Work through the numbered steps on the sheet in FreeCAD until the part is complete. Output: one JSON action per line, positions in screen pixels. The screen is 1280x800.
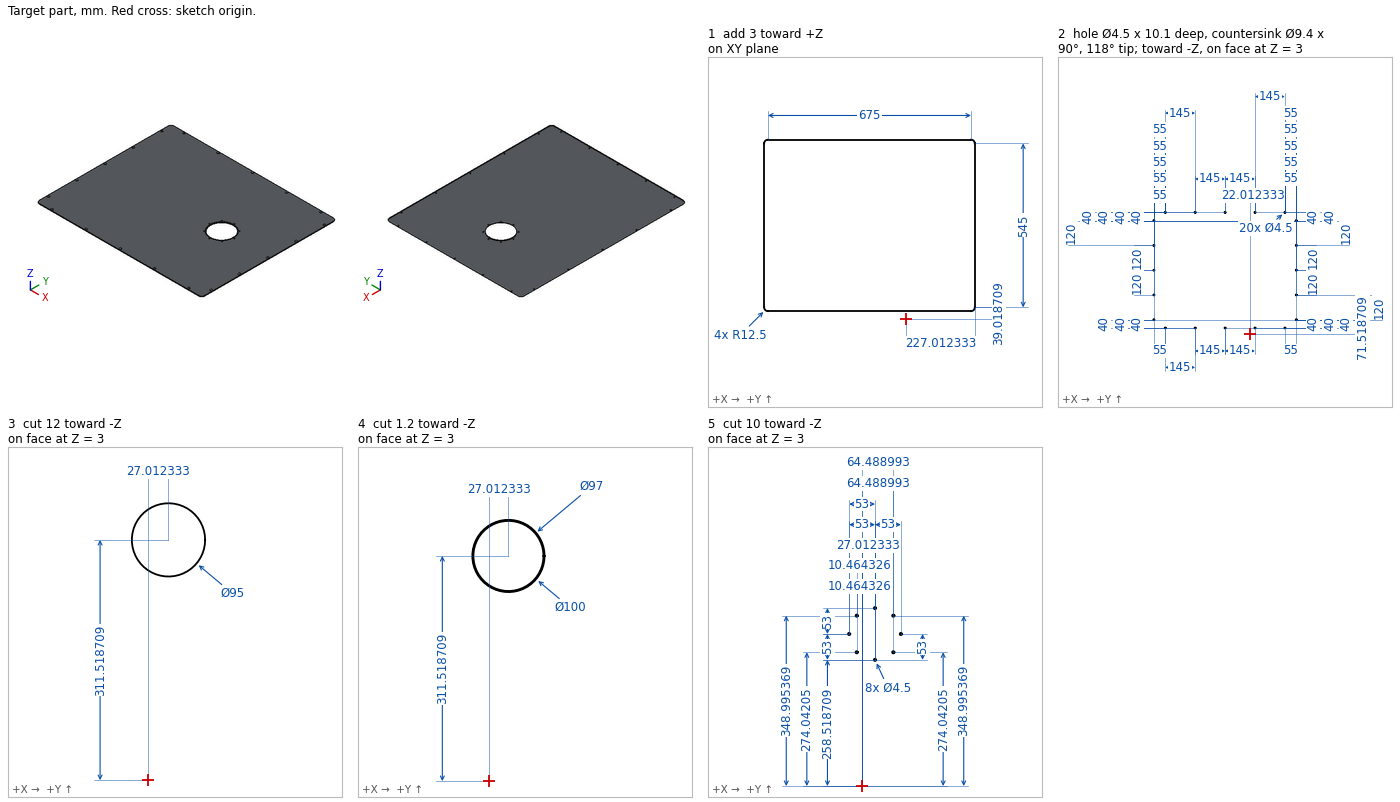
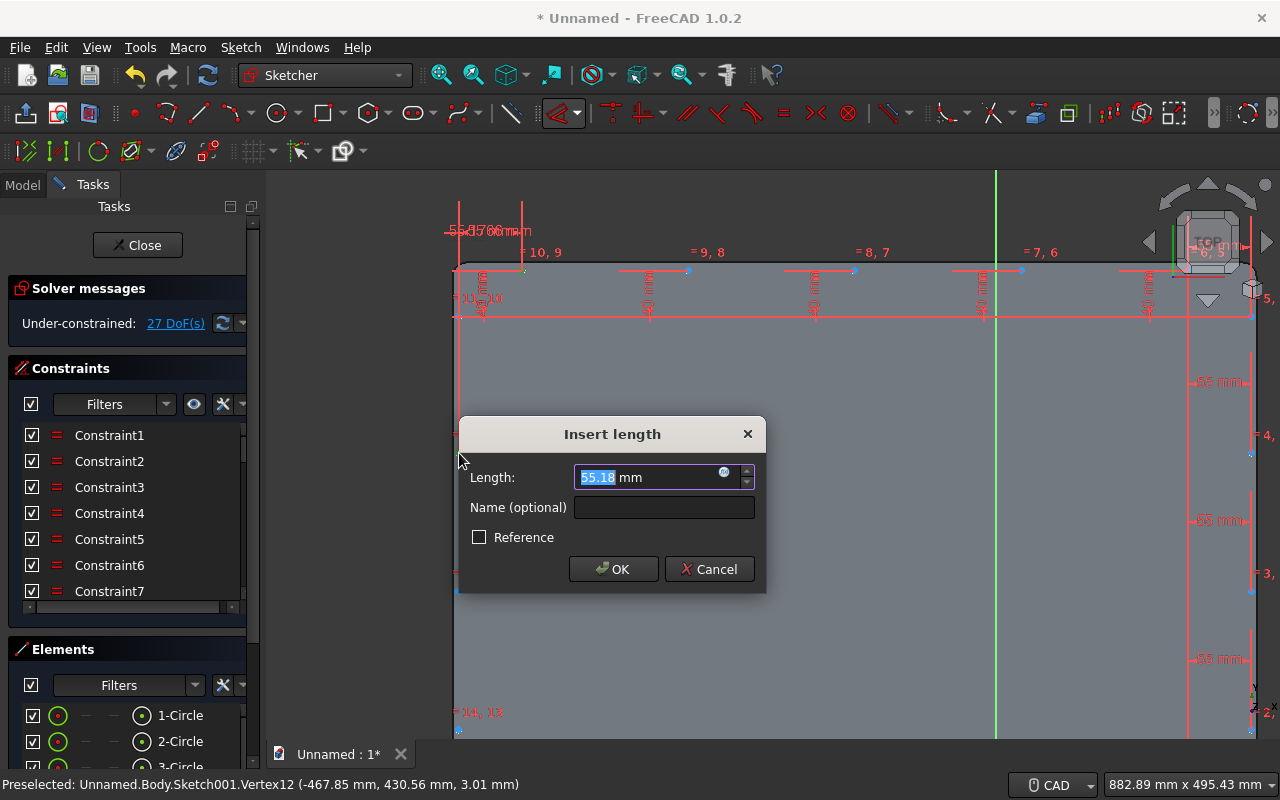
{"action": "type", "text": "55"}
{"action": "key", "text": "Return"}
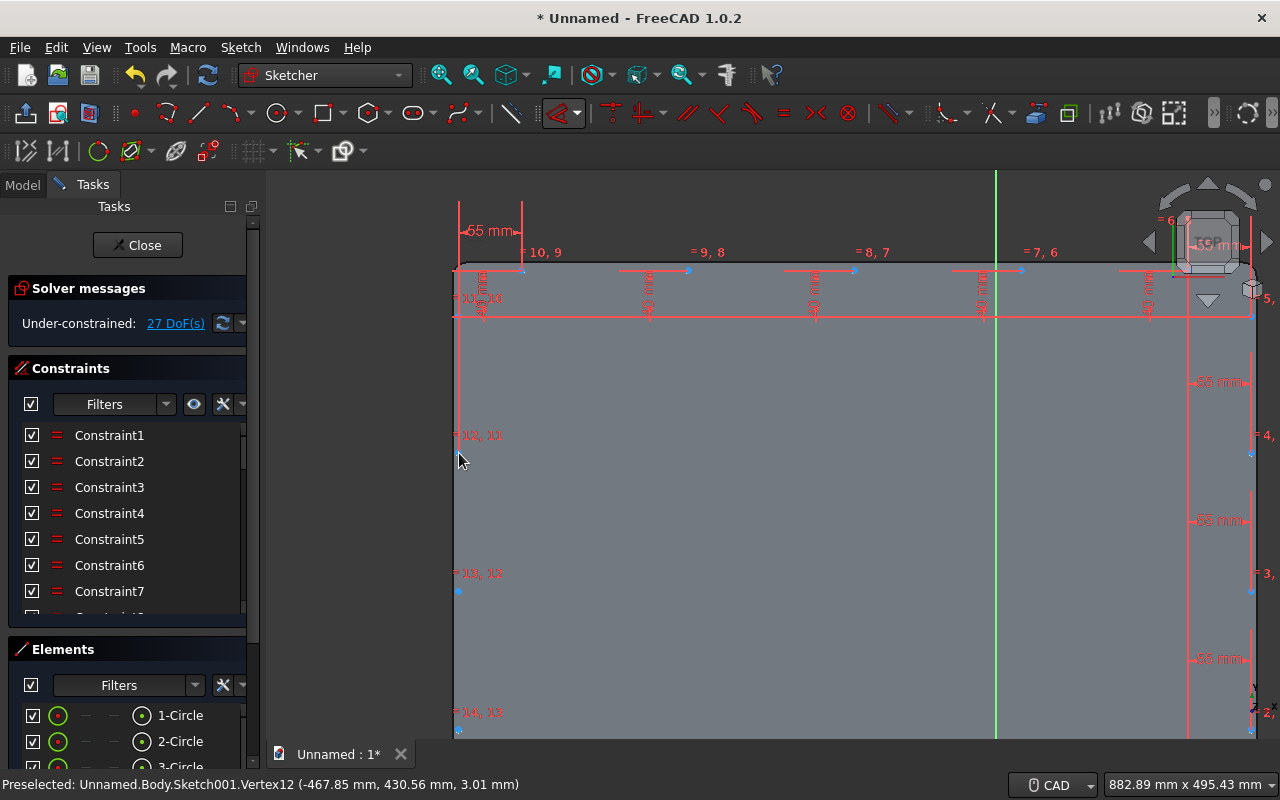
{"action": "left_click", "coordinate": [522, 271]}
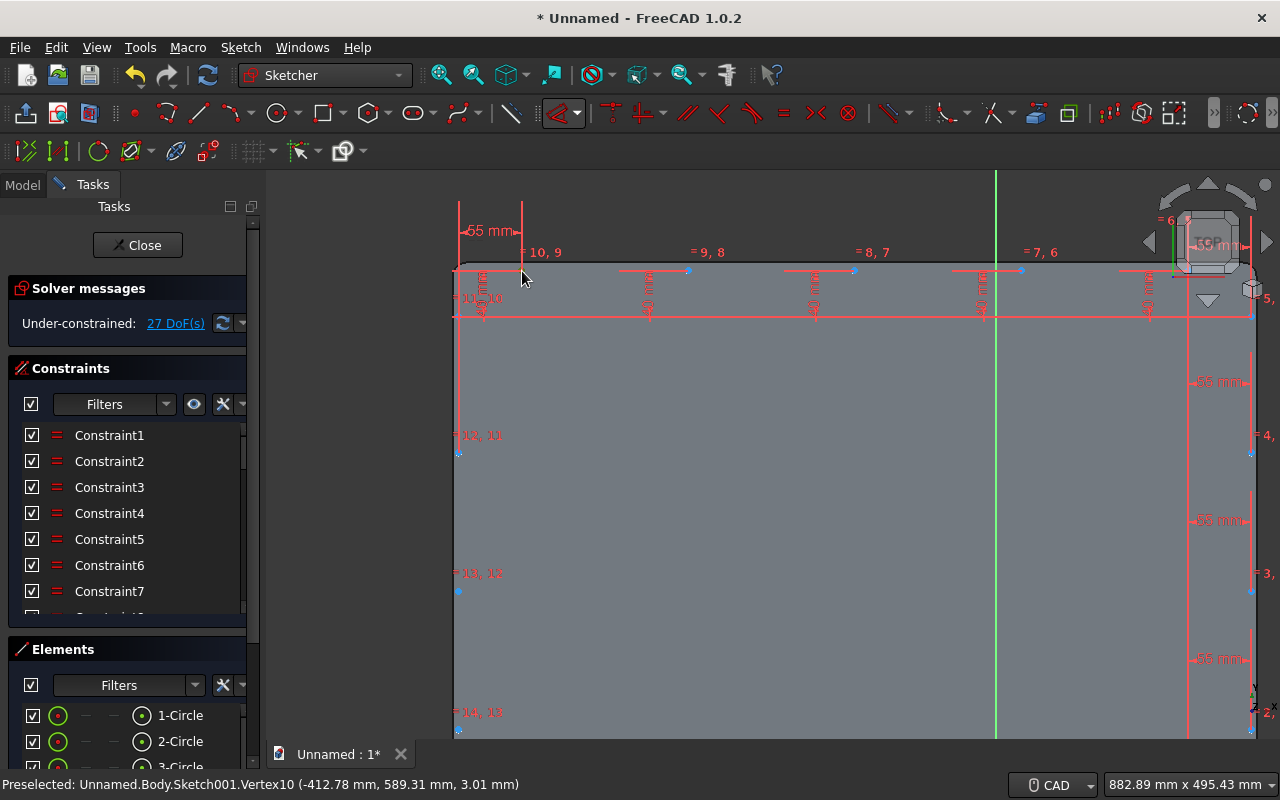
{"action": "left_click", "coordinate": [459, 591]}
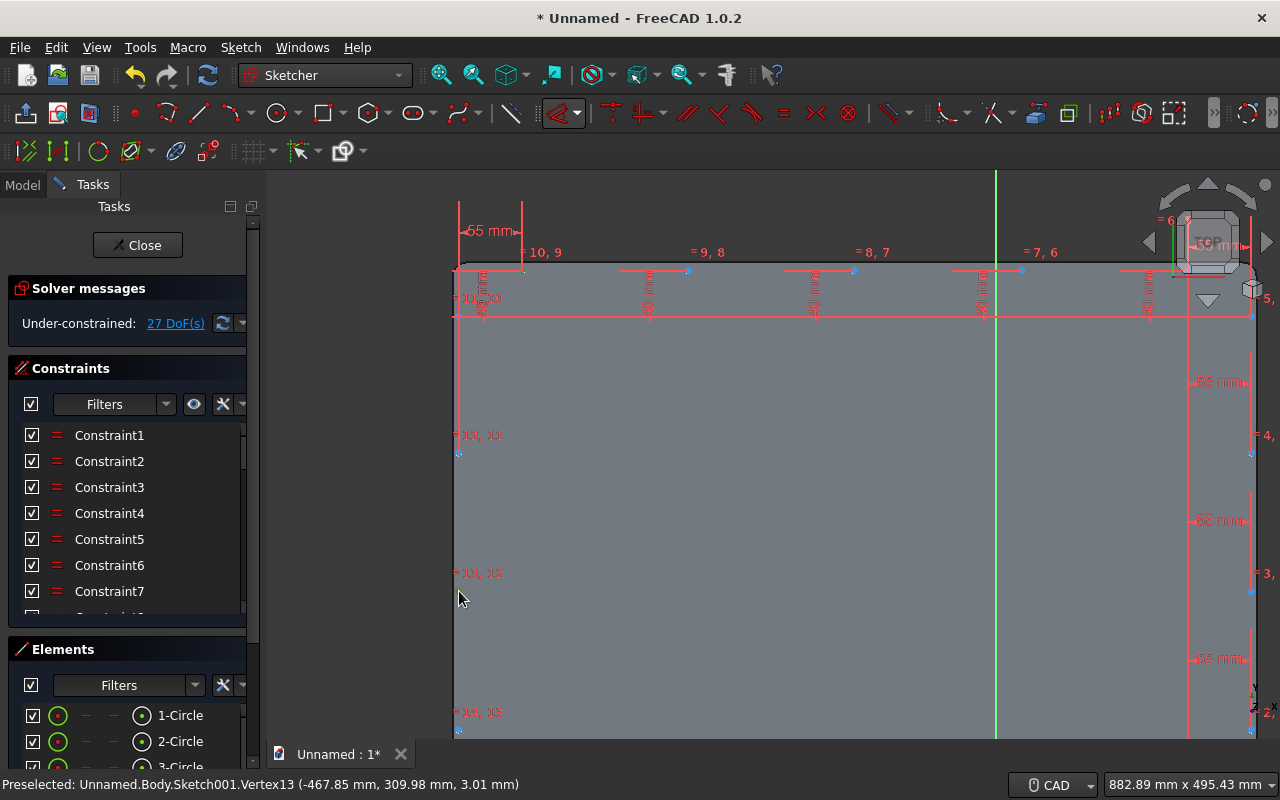
{"action": "left_click", "coordinate": [580, 114]}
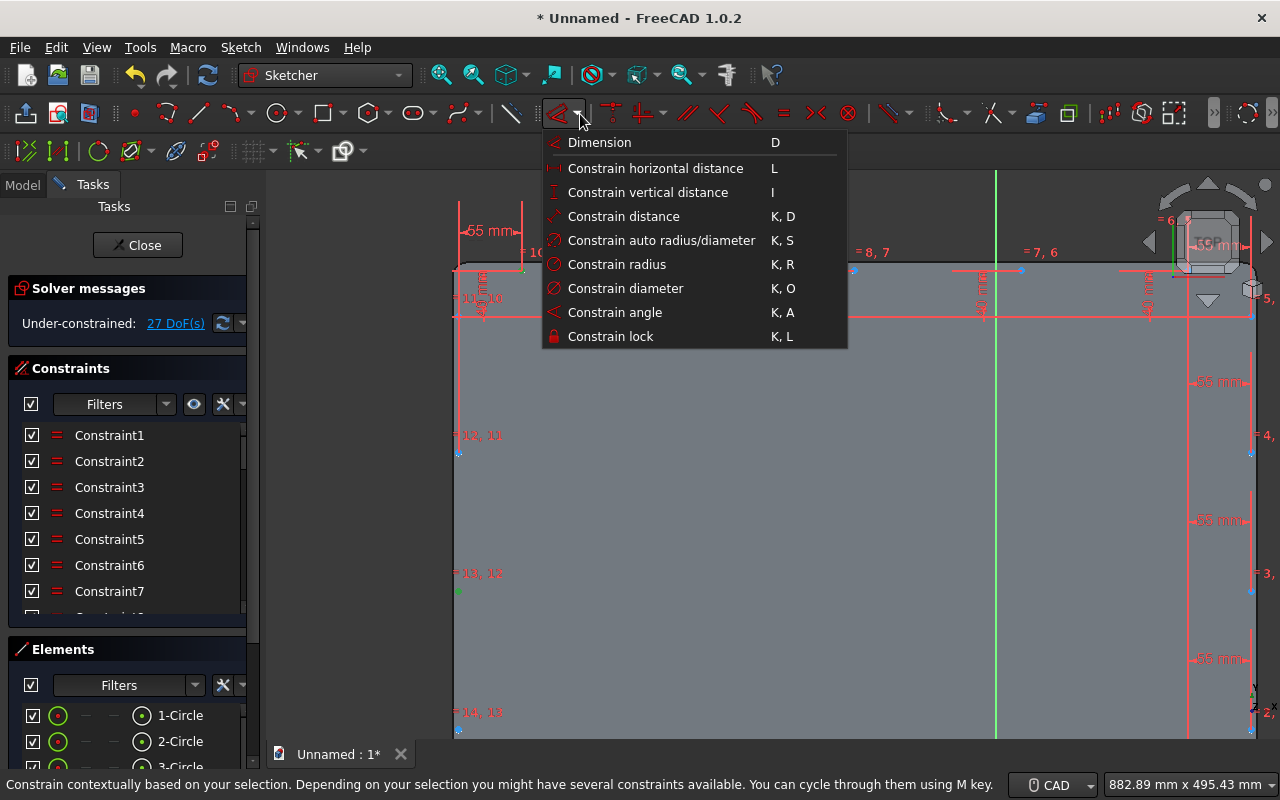
{"action": "left_click", "coordinate": [695, 168]}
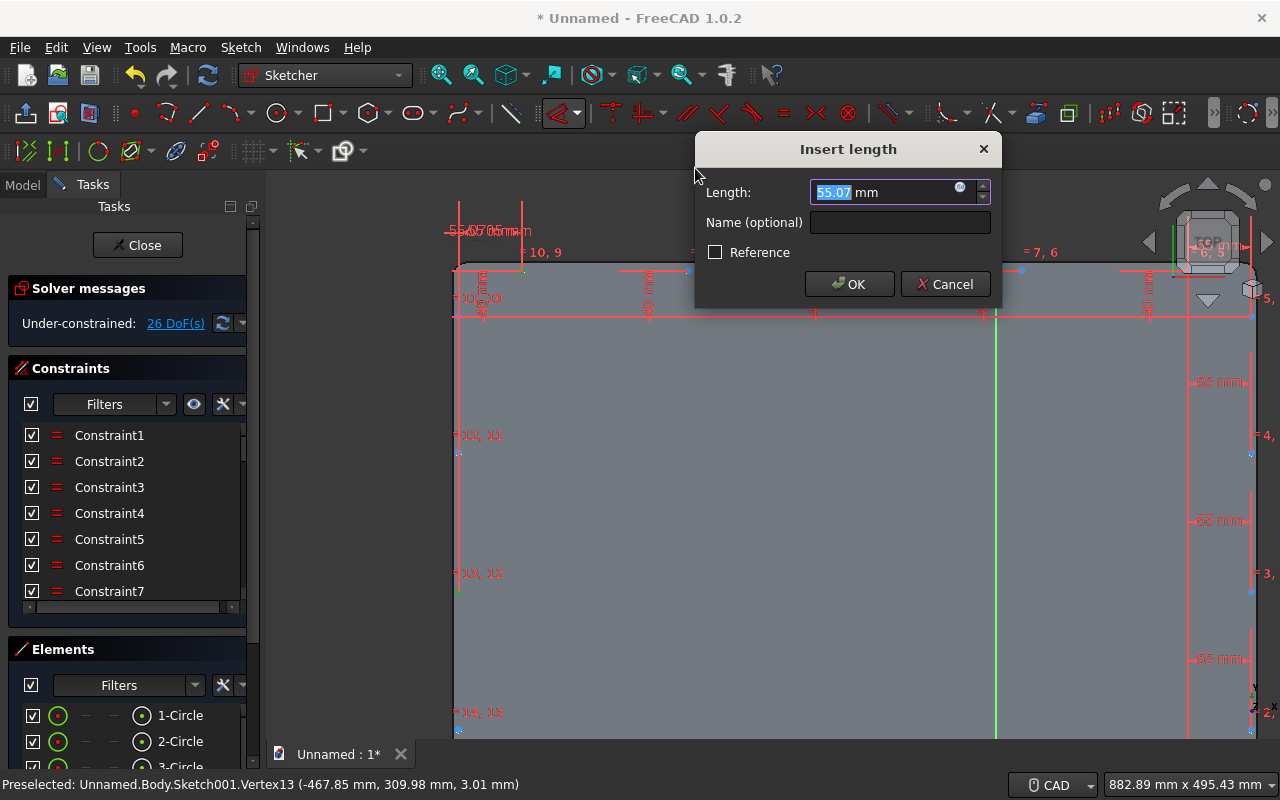
{"action": "type", "text": "55"}
{"action": "key", "text": "Return"}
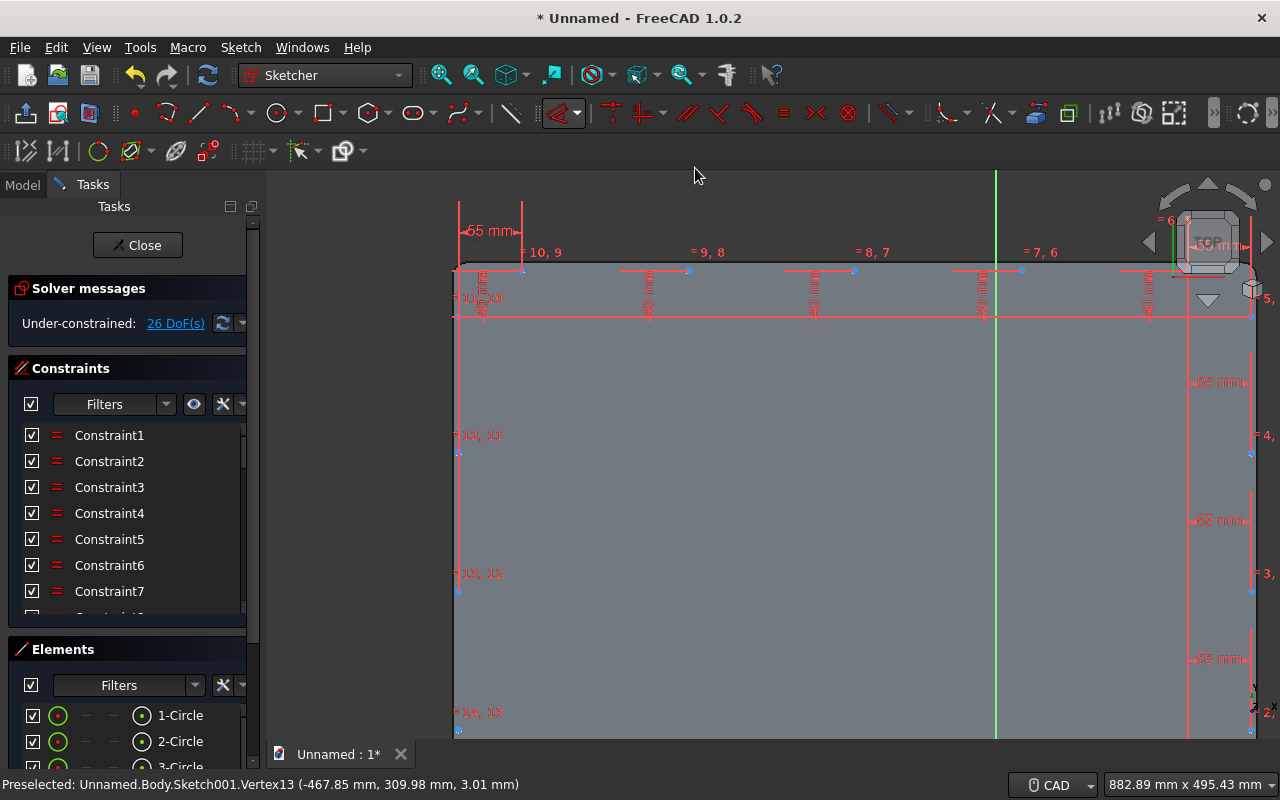
{"action": "left_click", "coordinate": [522, 271]}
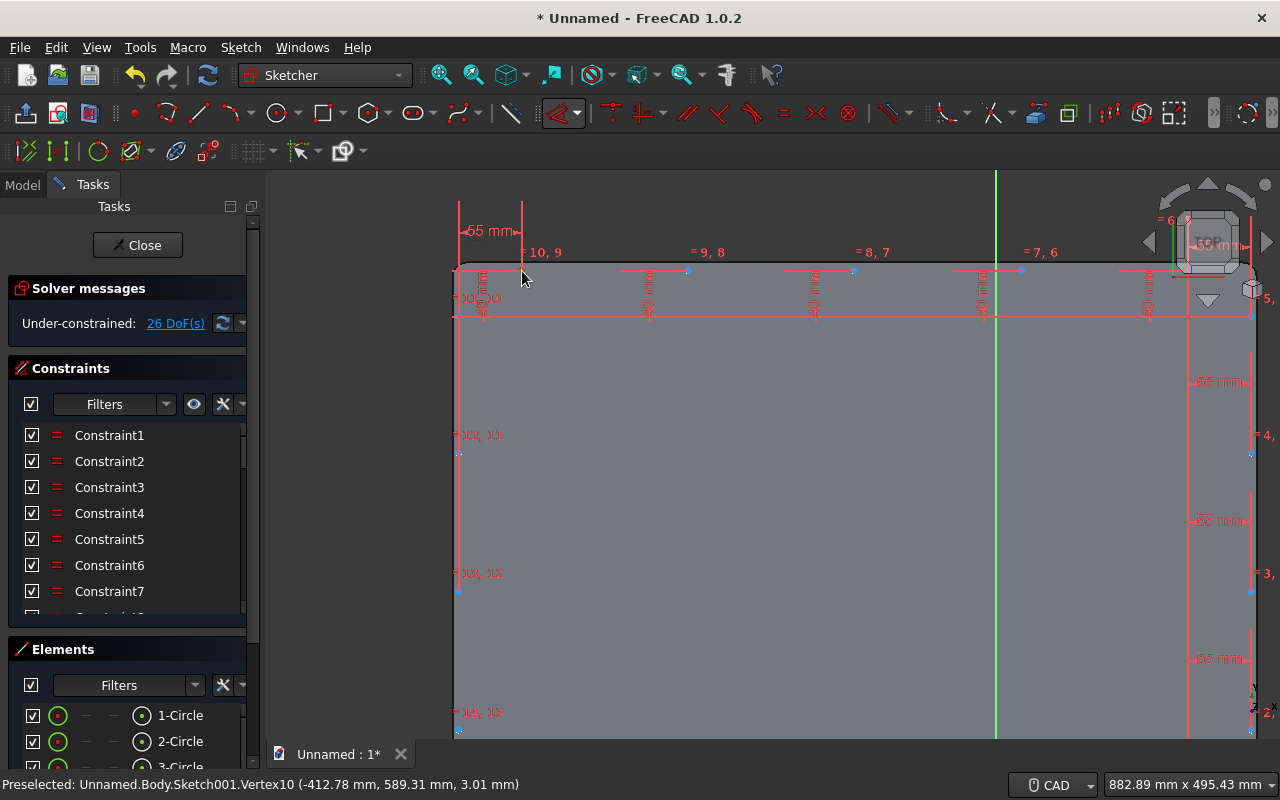
{"action": "scroll", "coordinate": [522, 270], "scroll_direction": "down", "scroll_amount": 3}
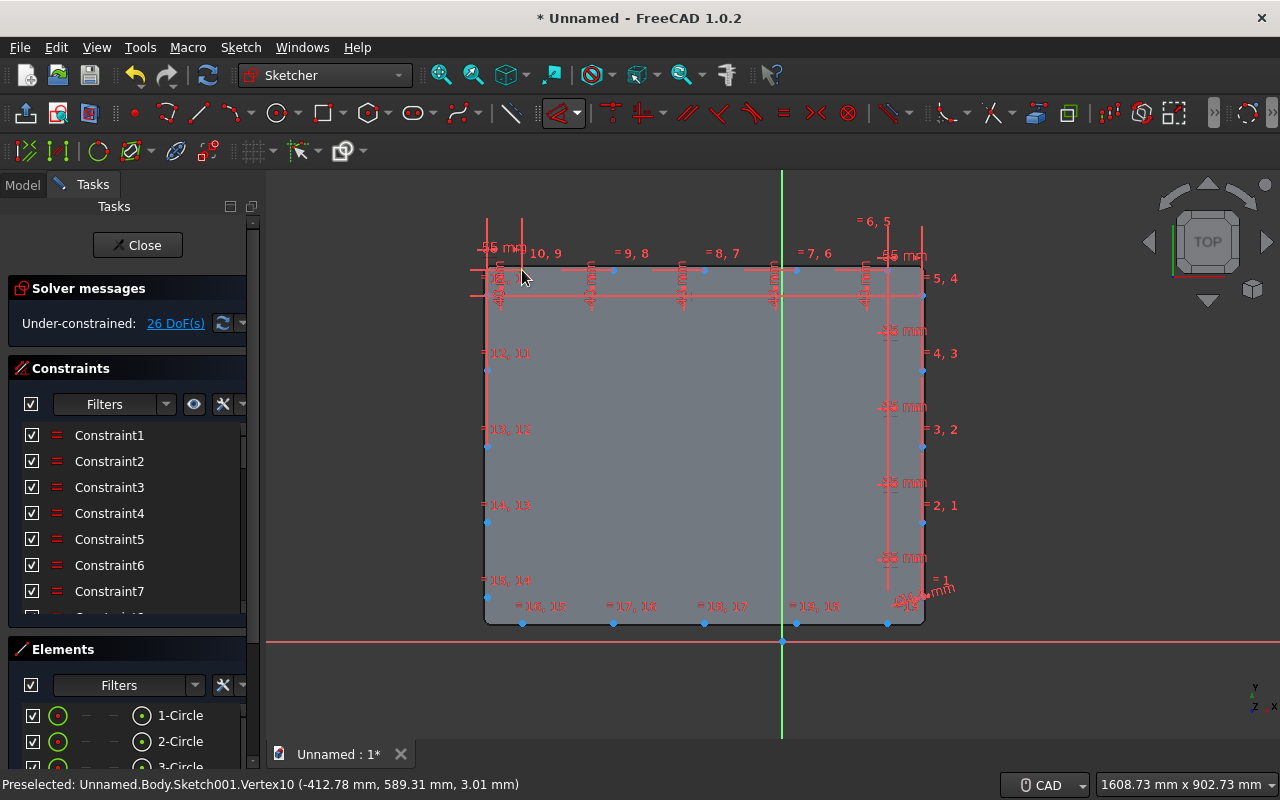
{"action": "left_click", "coordinate": [487, 522]}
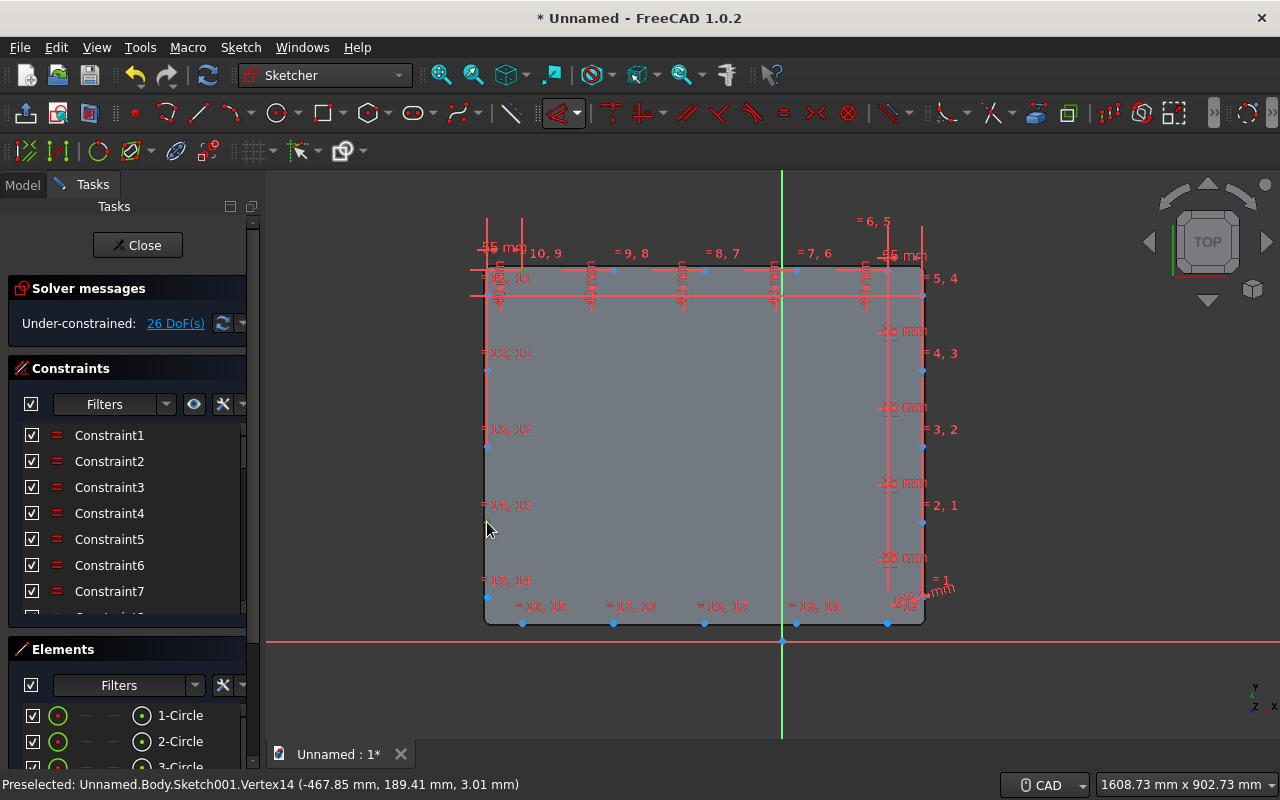
{"action": "left_click", "coordinate": [580, 114]}